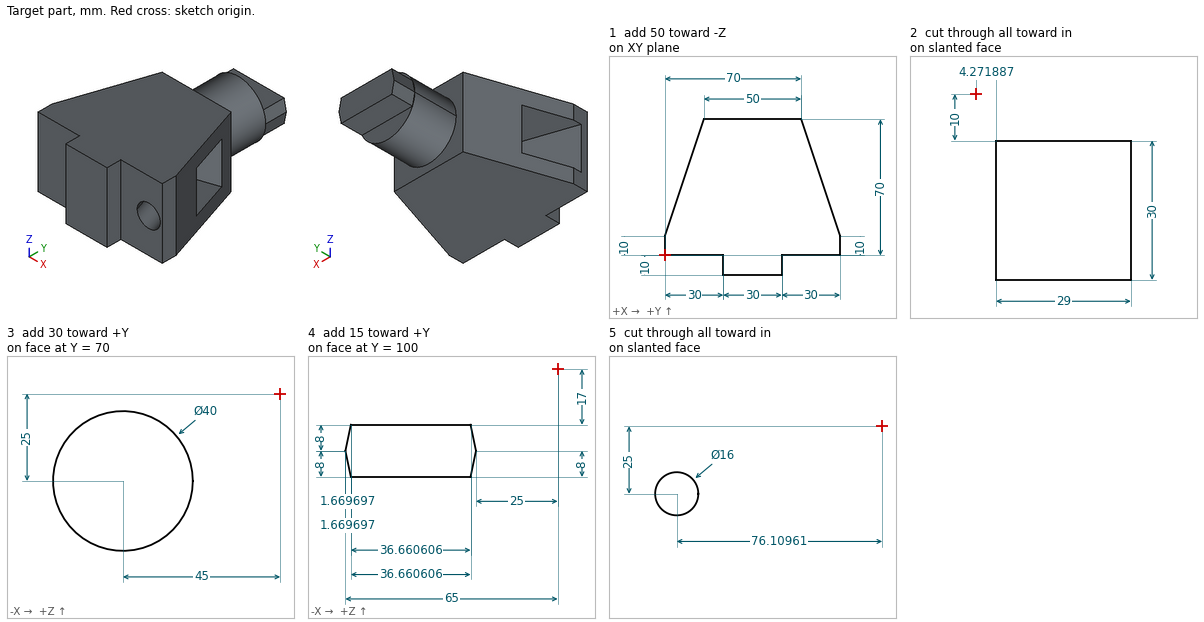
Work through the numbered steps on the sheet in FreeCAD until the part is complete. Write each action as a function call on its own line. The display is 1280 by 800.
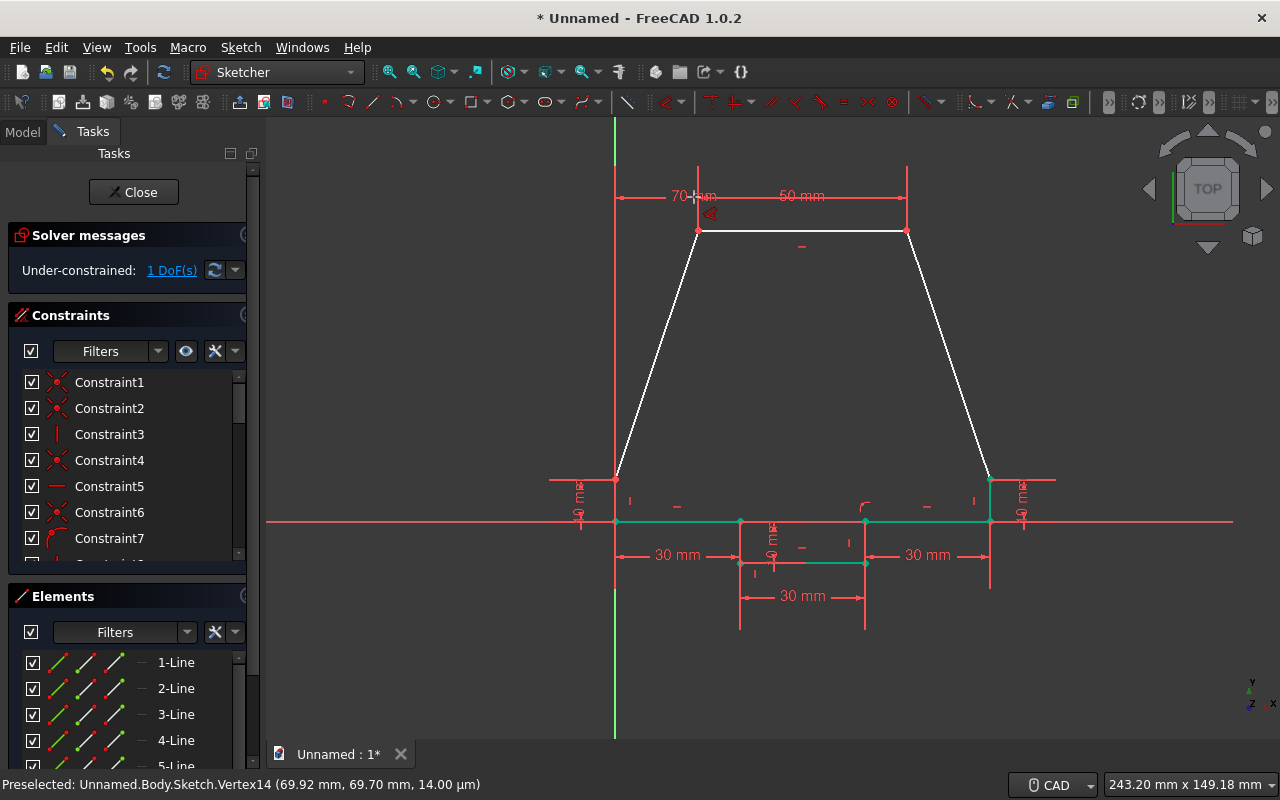
click(907, 231)
click(581, 376)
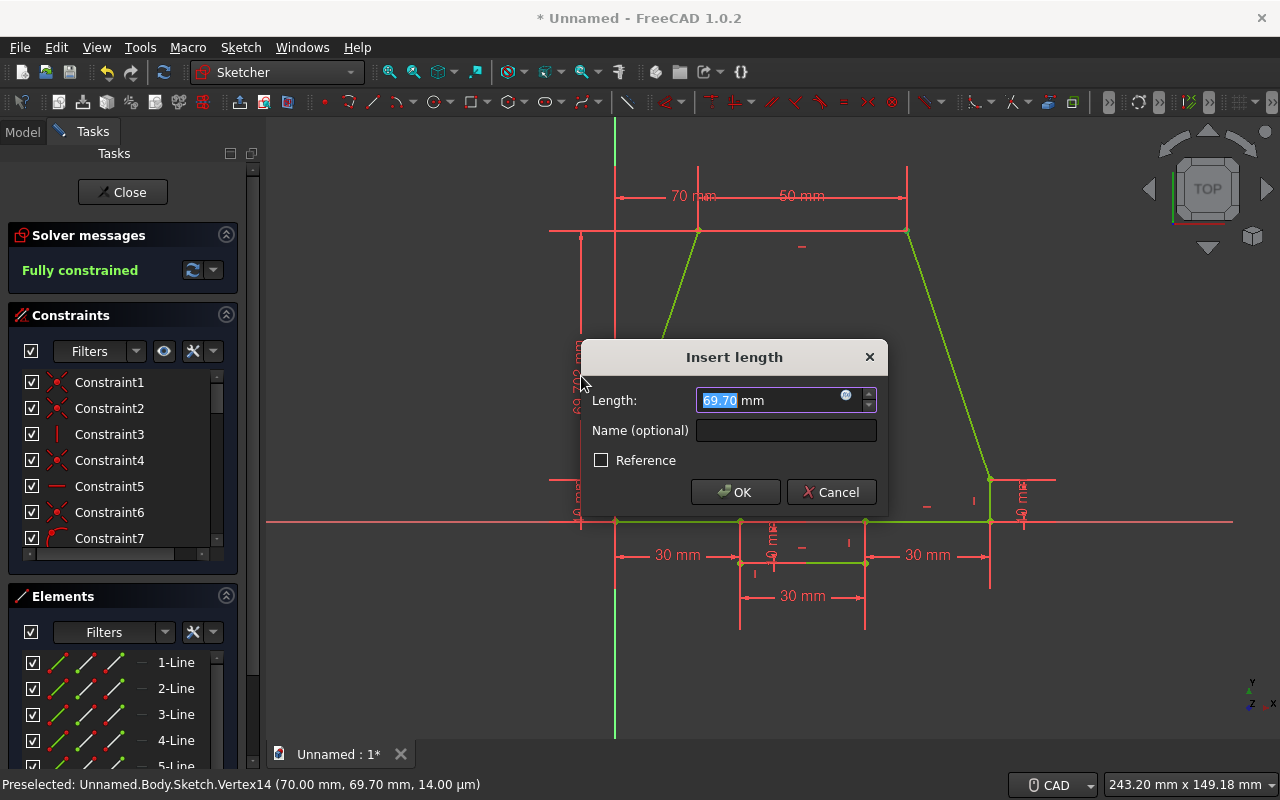
text(70)
key(Return)
key(Escape)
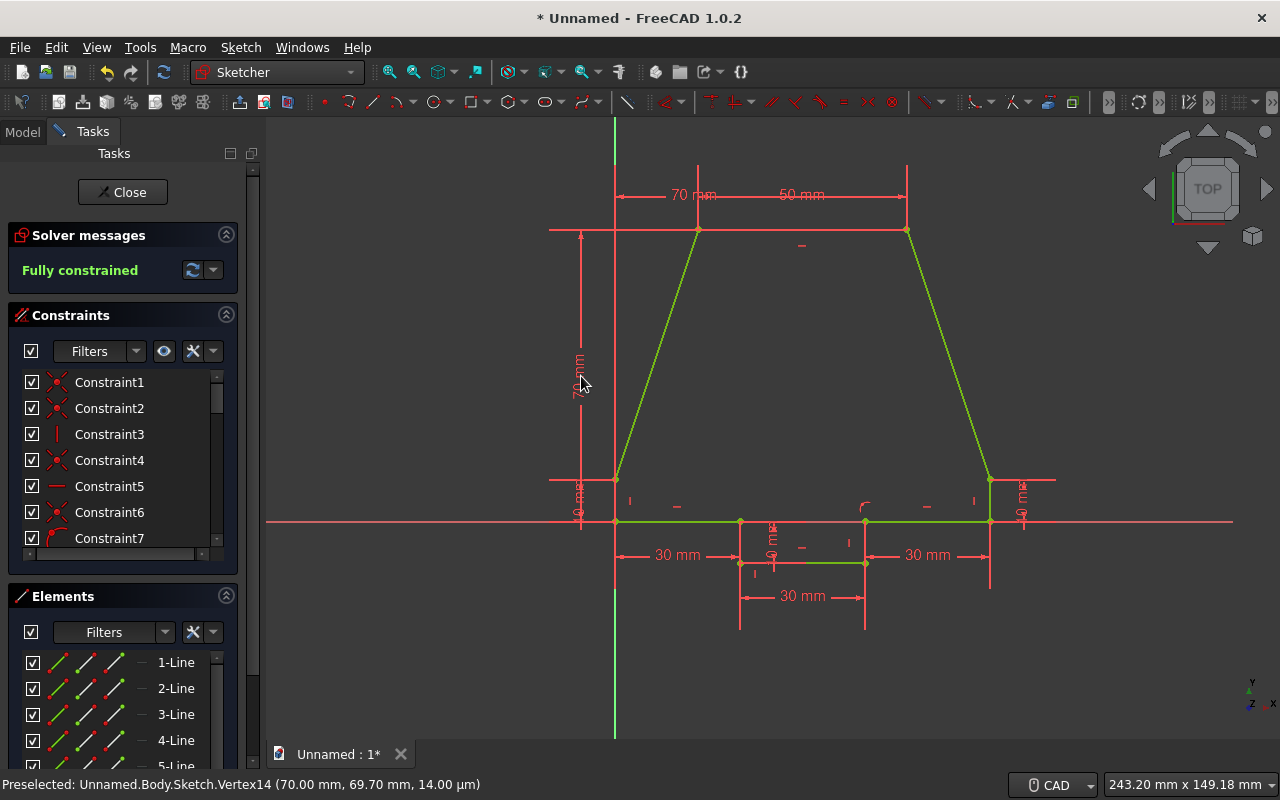
click(123, 192)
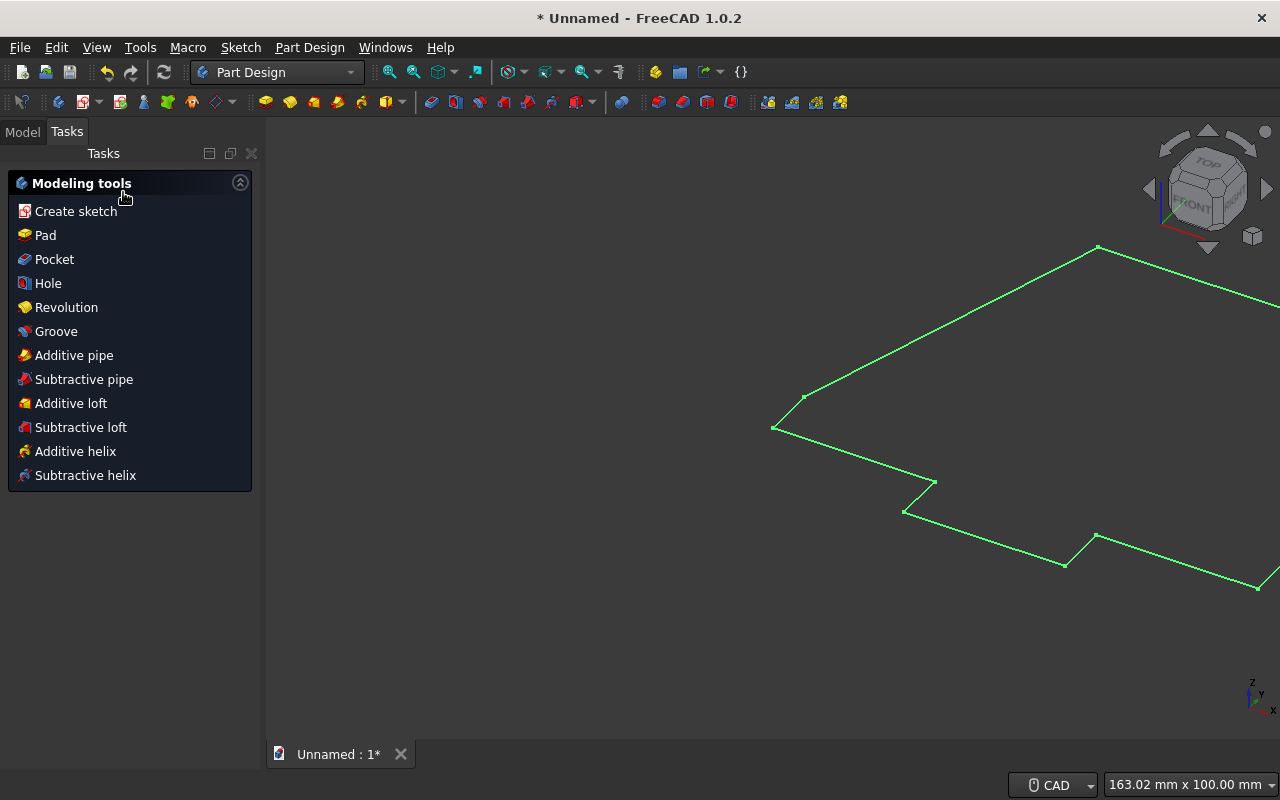
click(266, 102)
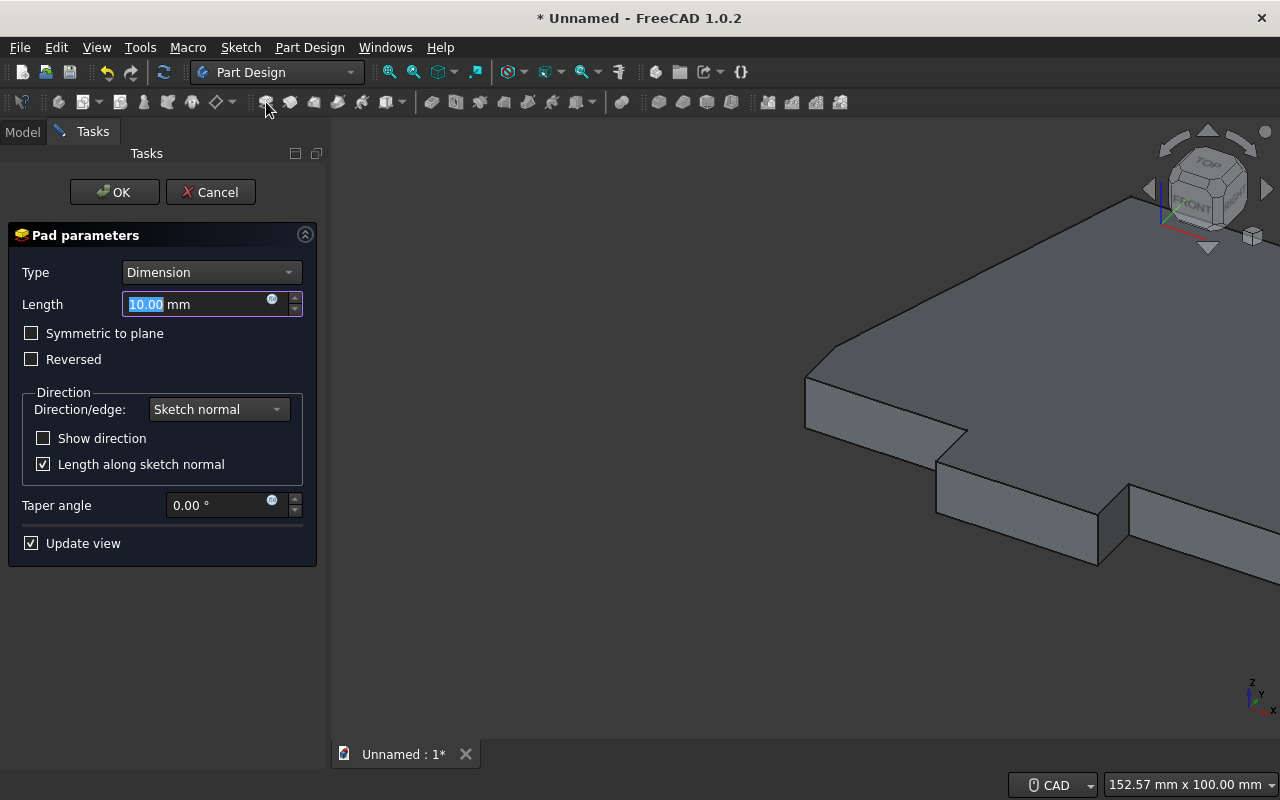
text(50)
key(Tab)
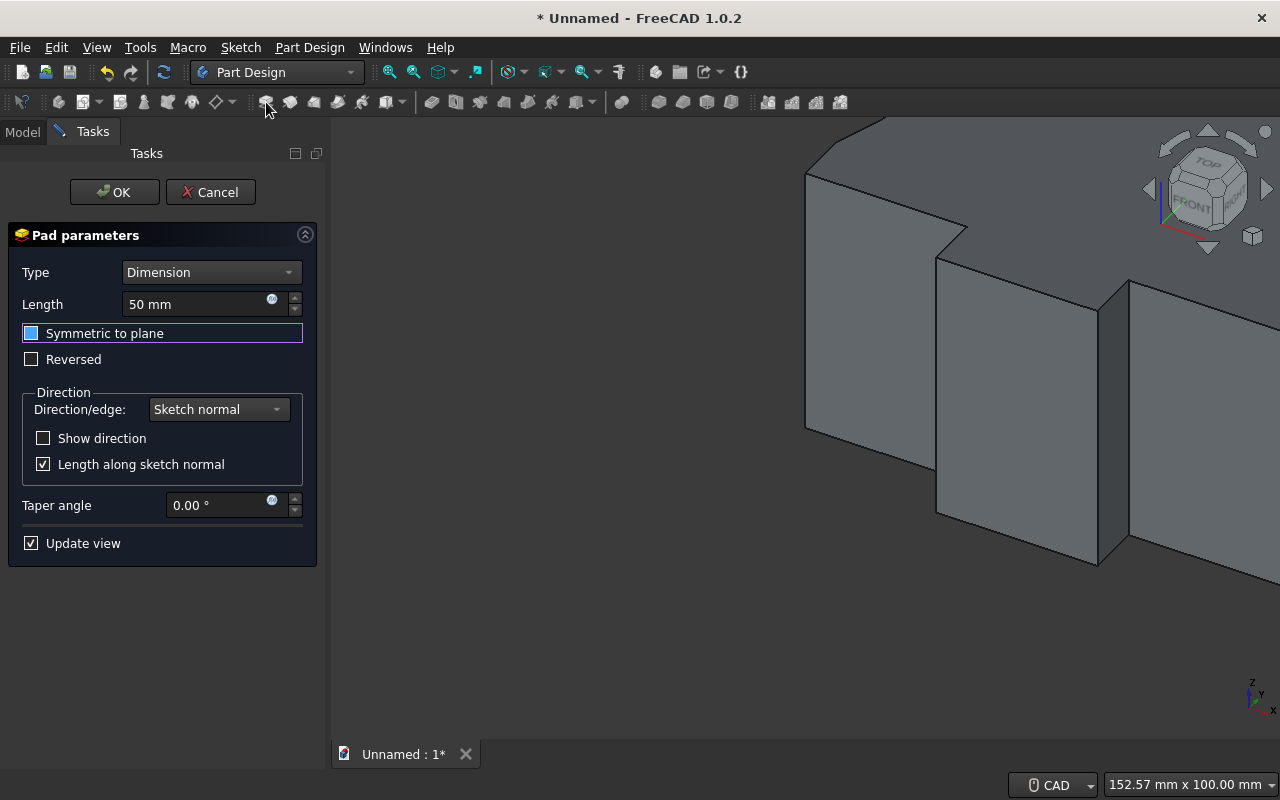
click(30, 359)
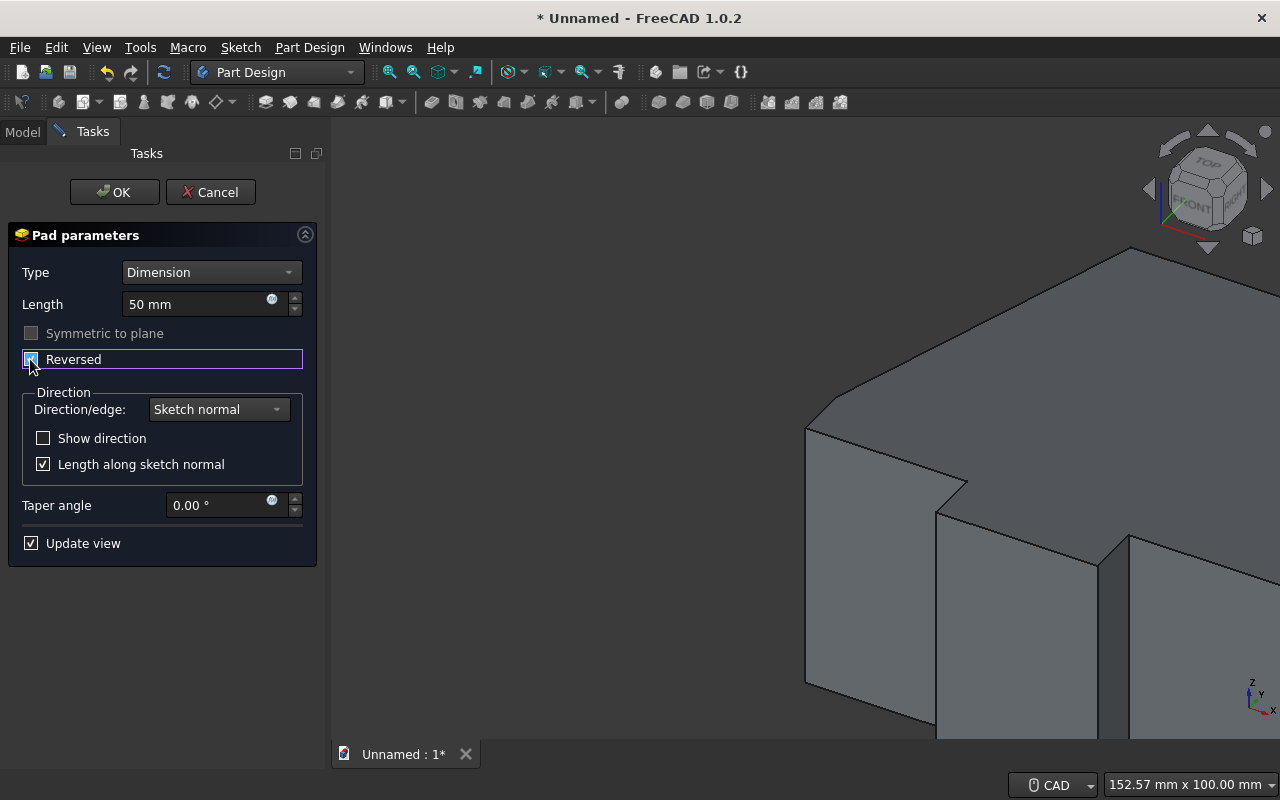
click(115, 192)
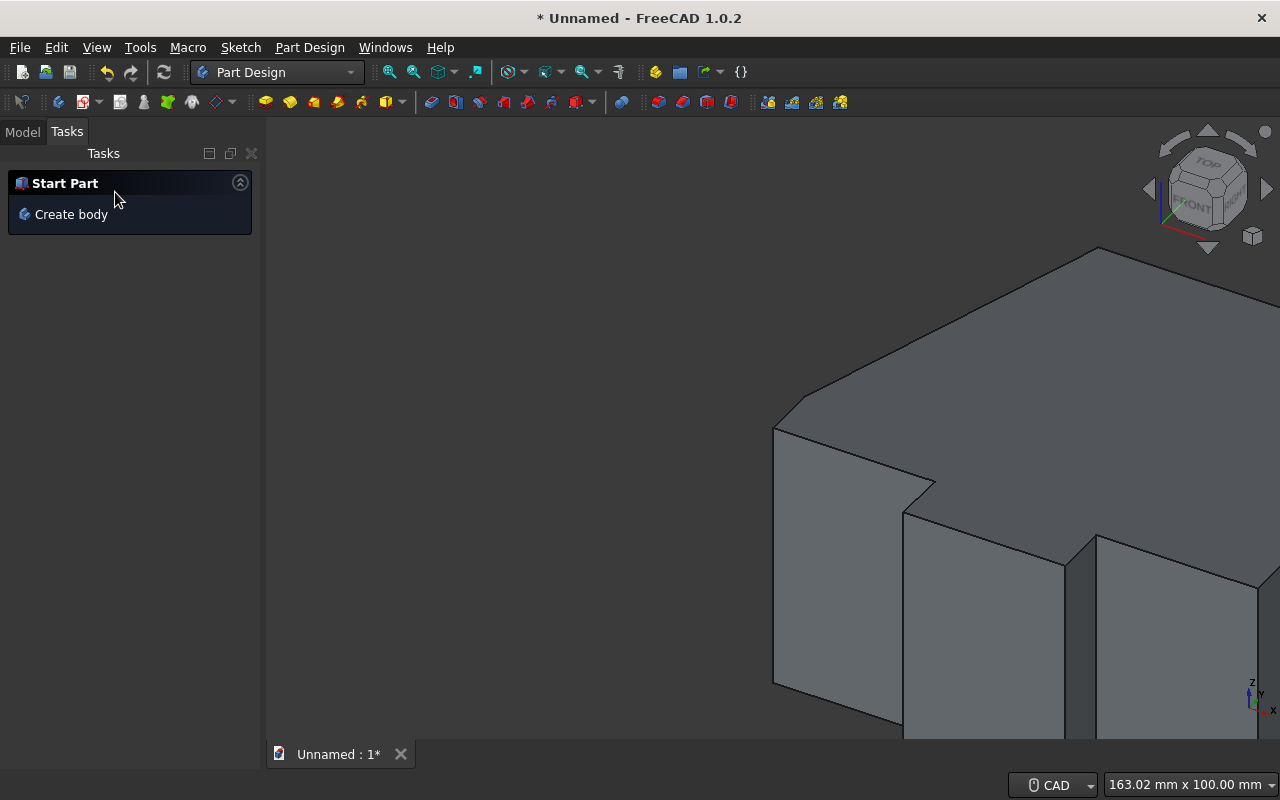
key(v)
key(f)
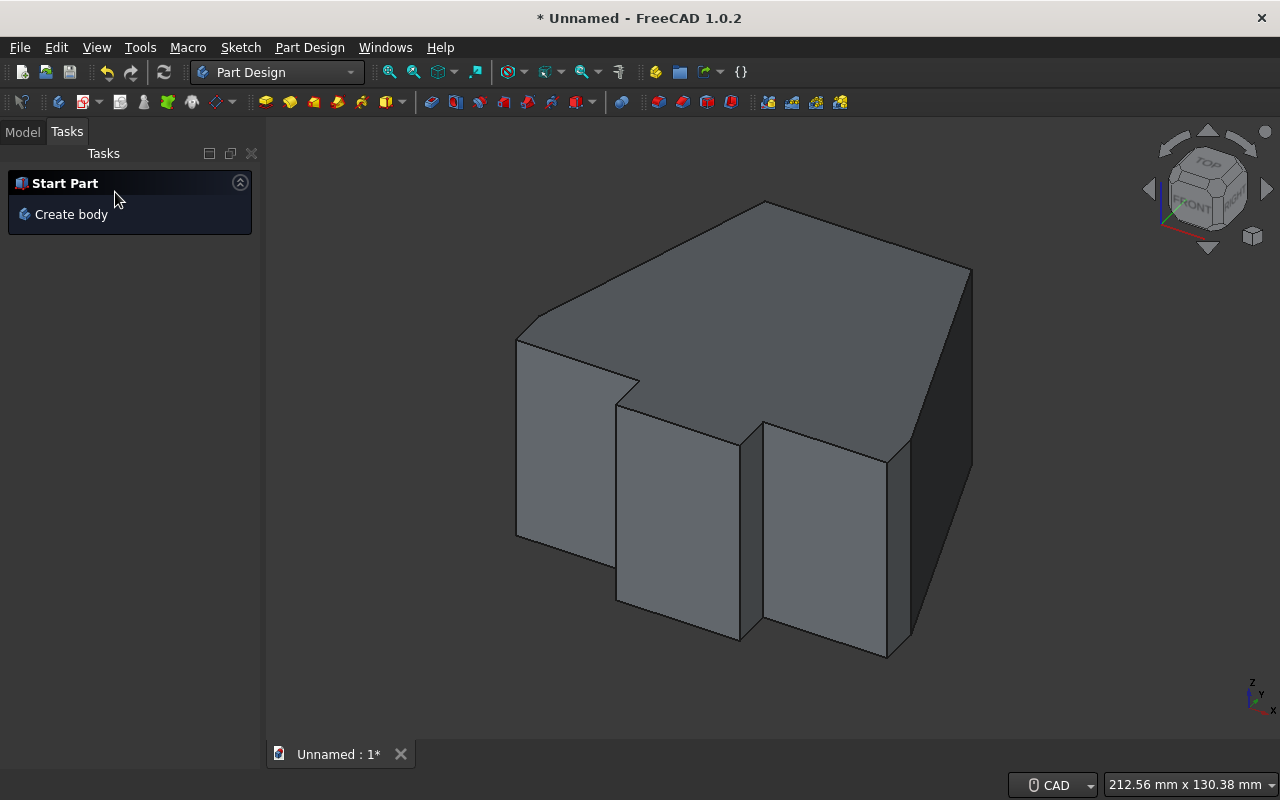
click(941, 451)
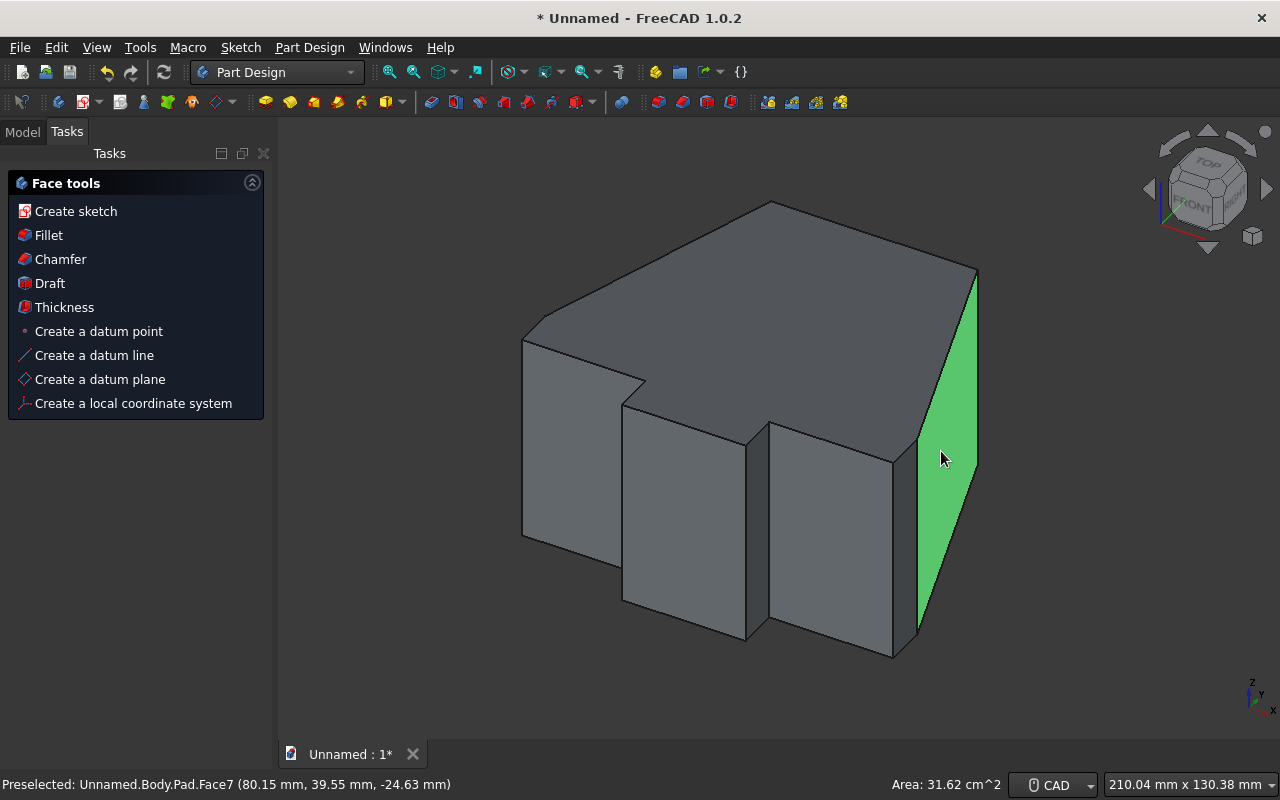
click(84, 102)